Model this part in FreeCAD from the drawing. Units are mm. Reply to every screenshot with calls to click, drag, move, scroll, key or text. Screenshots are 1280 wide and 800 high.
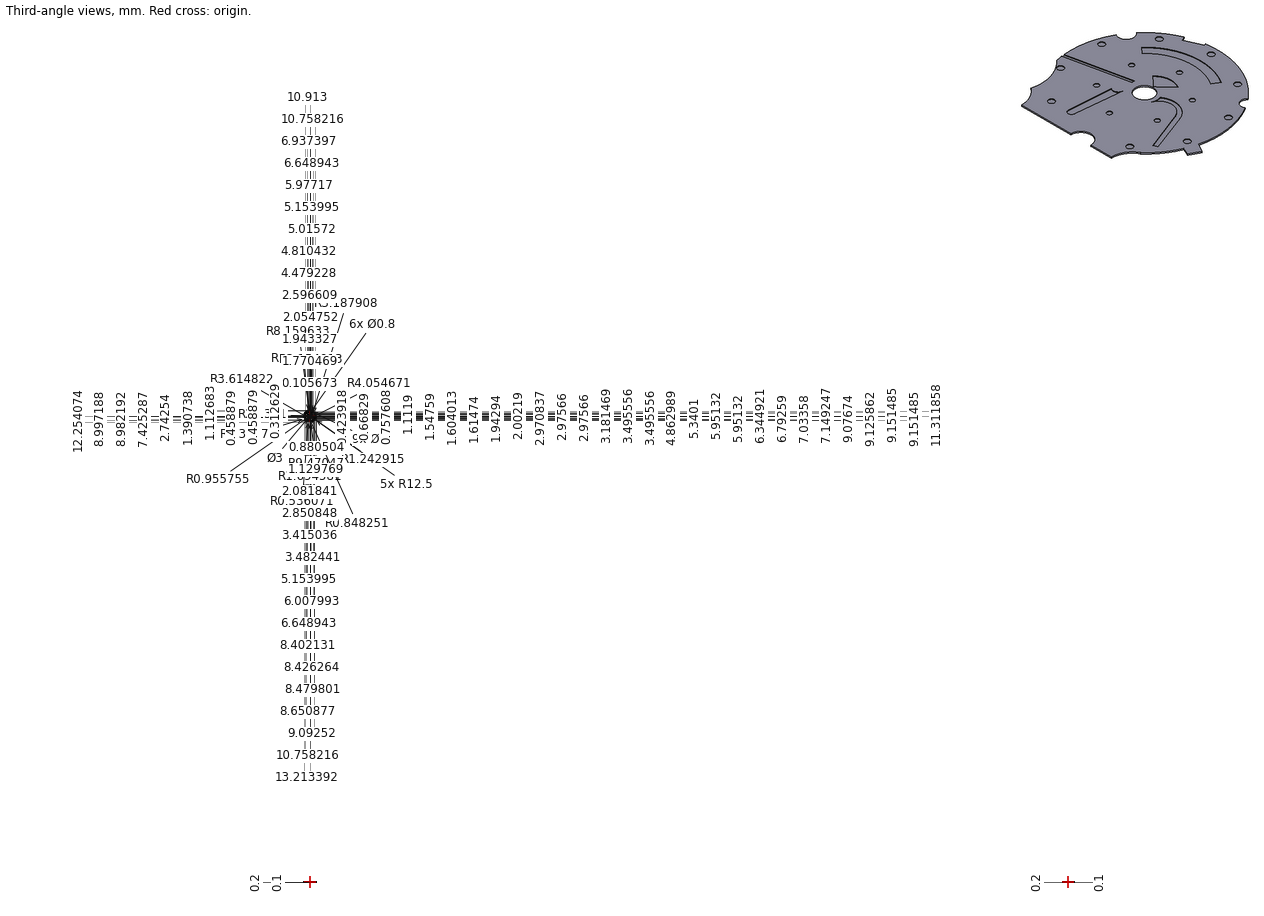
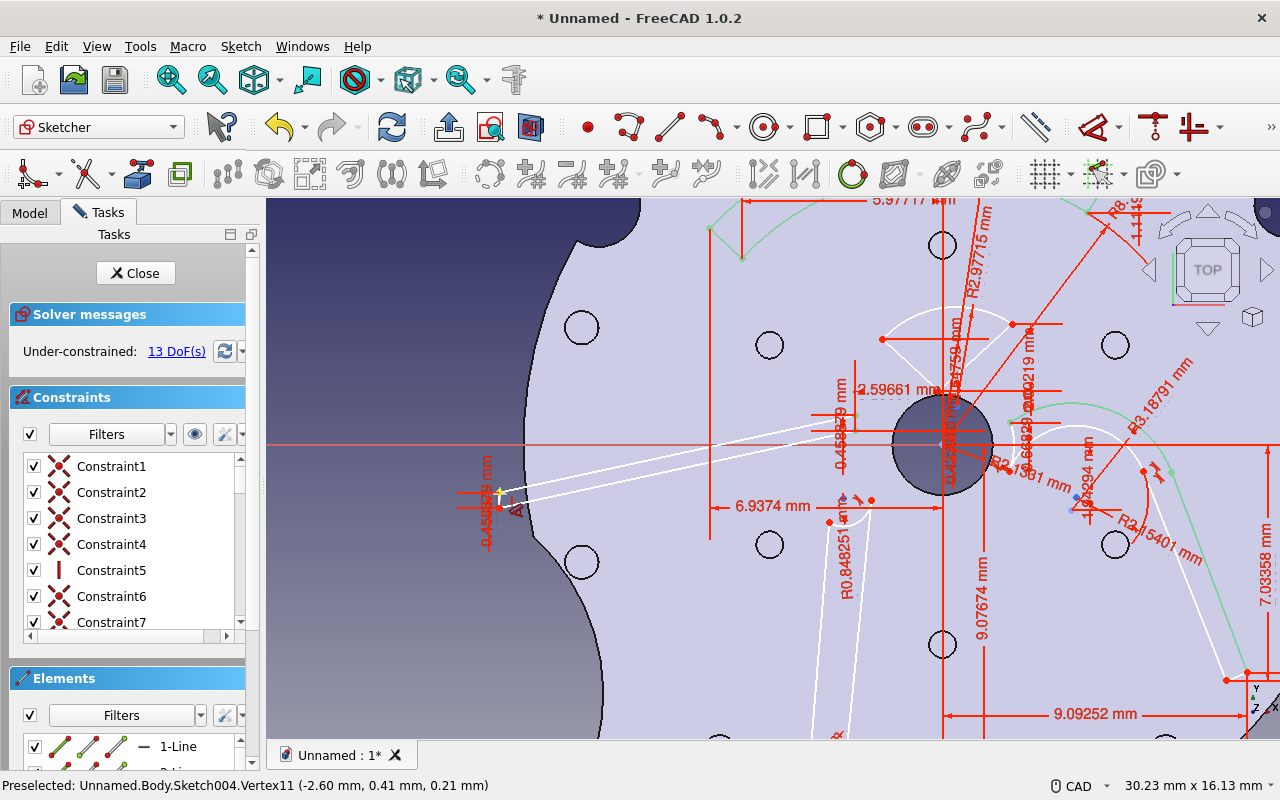
click(499, 493)
click(465, 469)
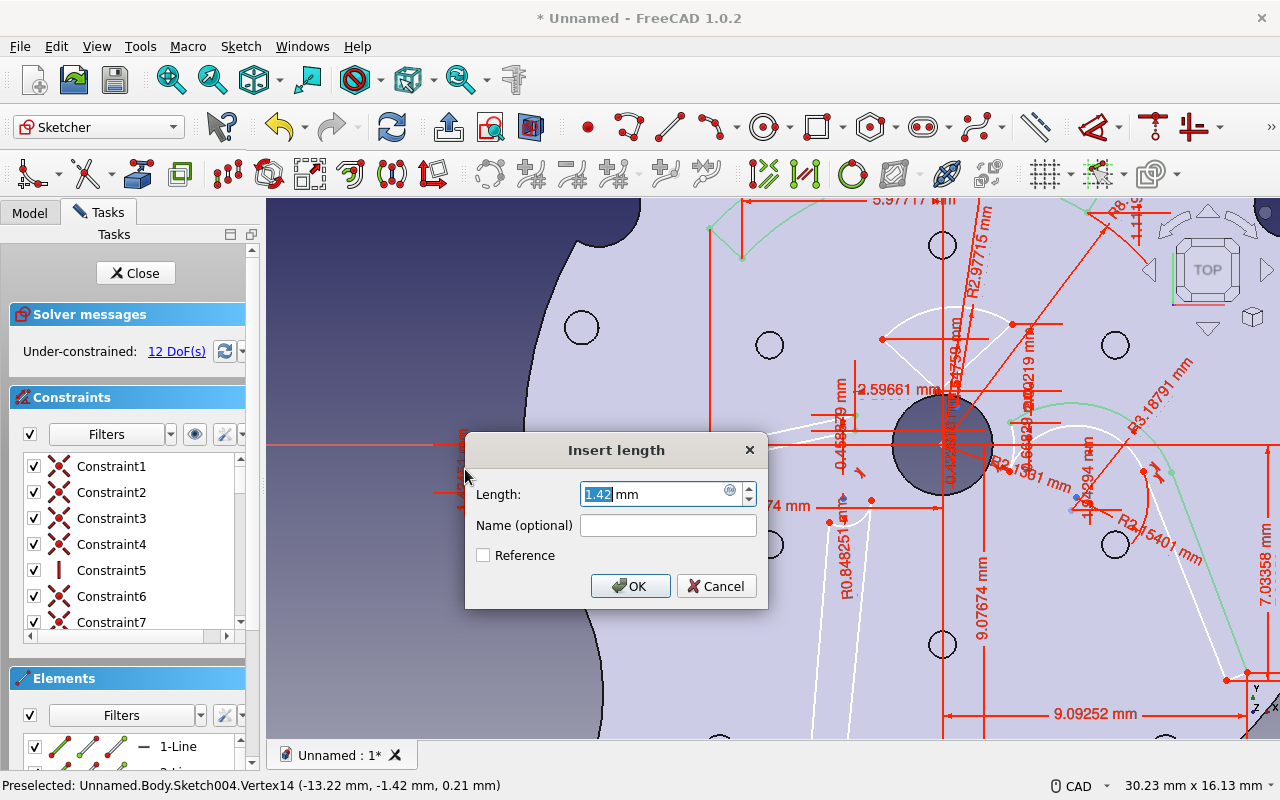
text(1.390738)
key(Return)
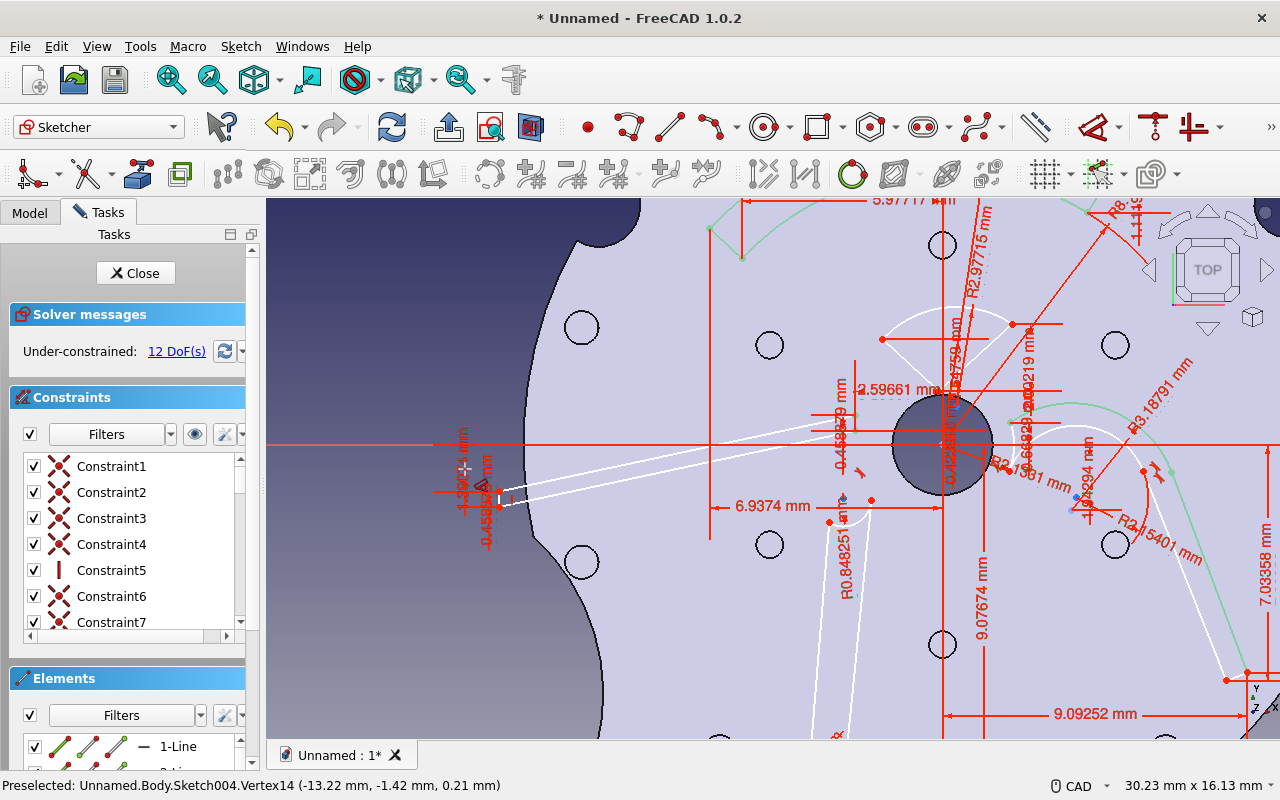
scroll(499, 493, down, 3)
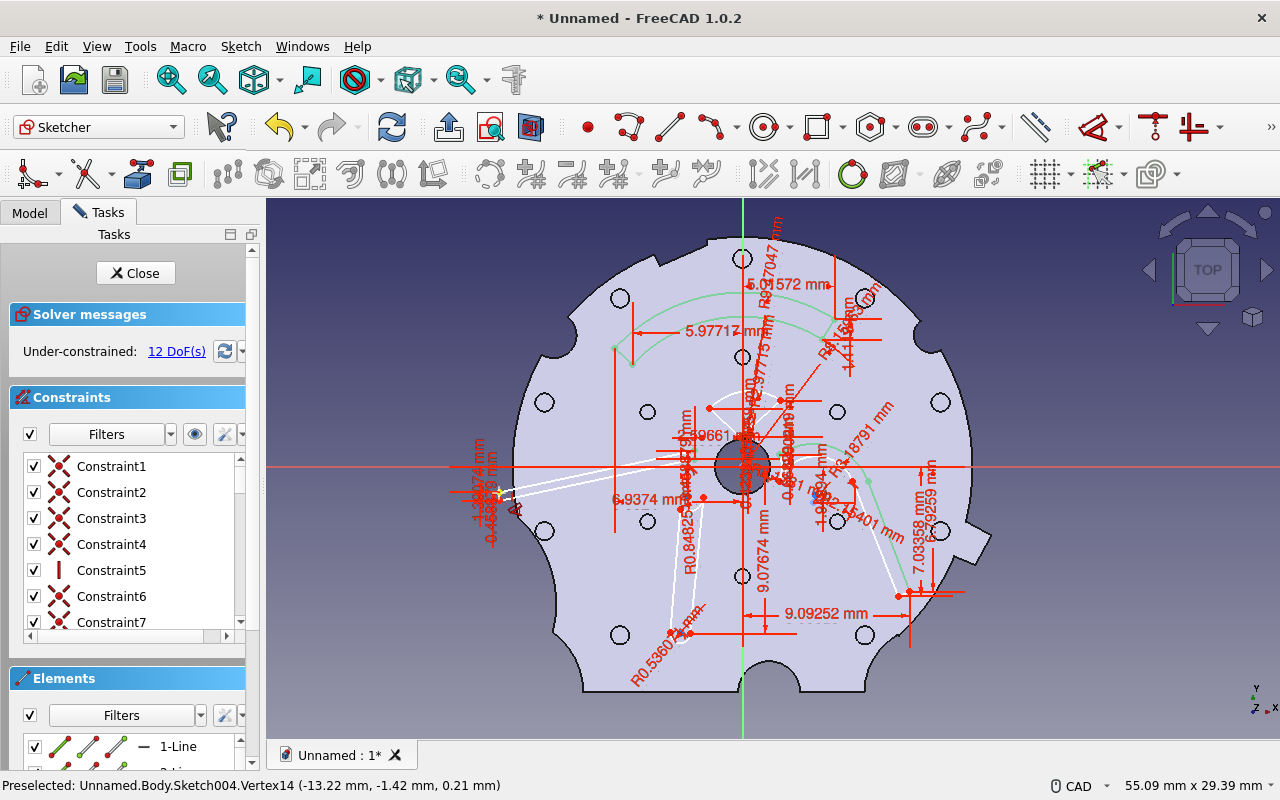
scroll(690, 634, up, 2)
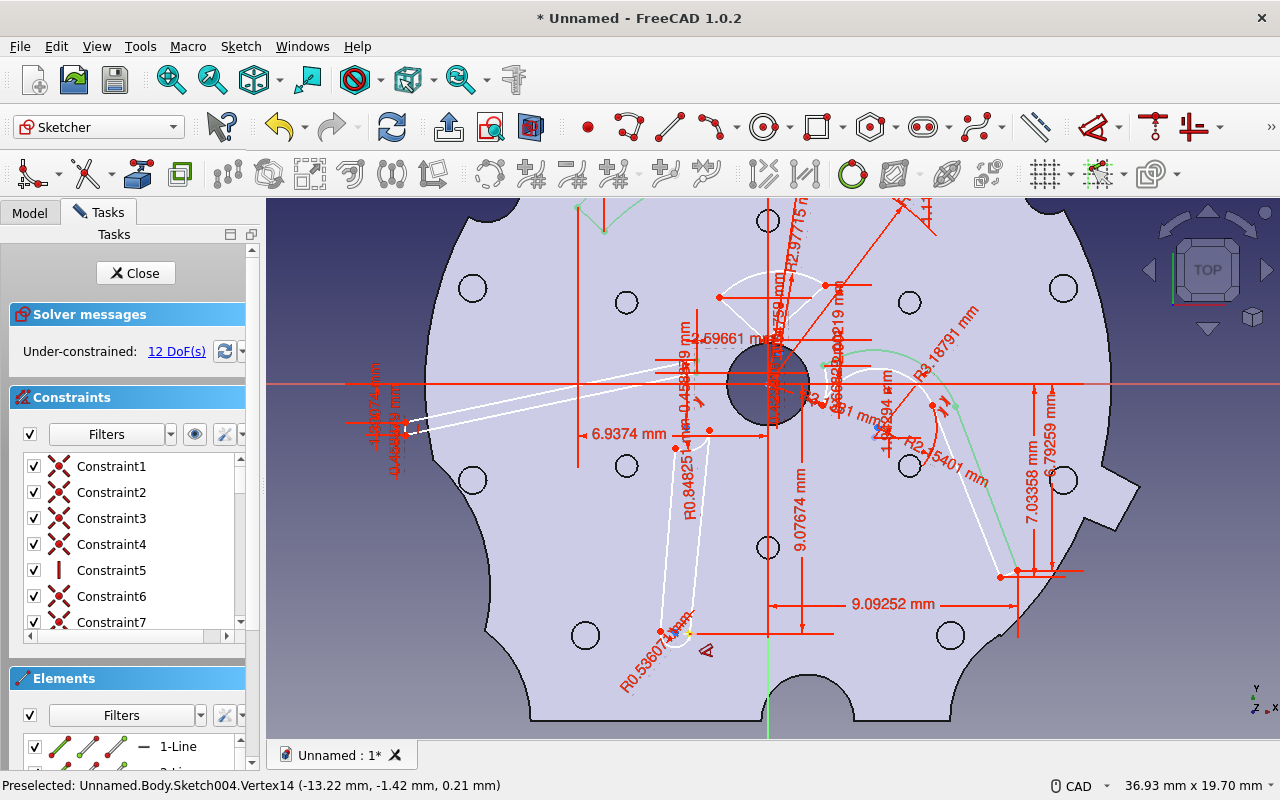
click(690, 634)
click(729, 668)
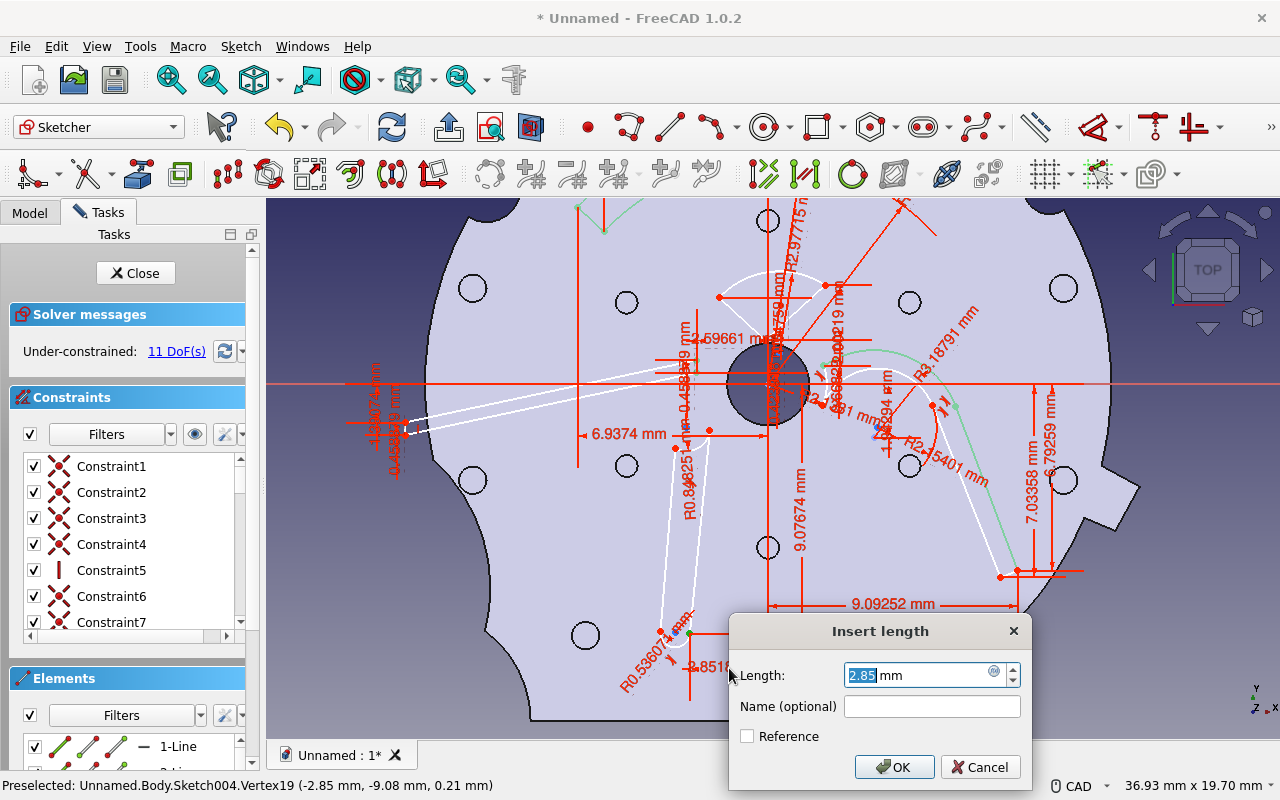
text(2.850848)
key(Return)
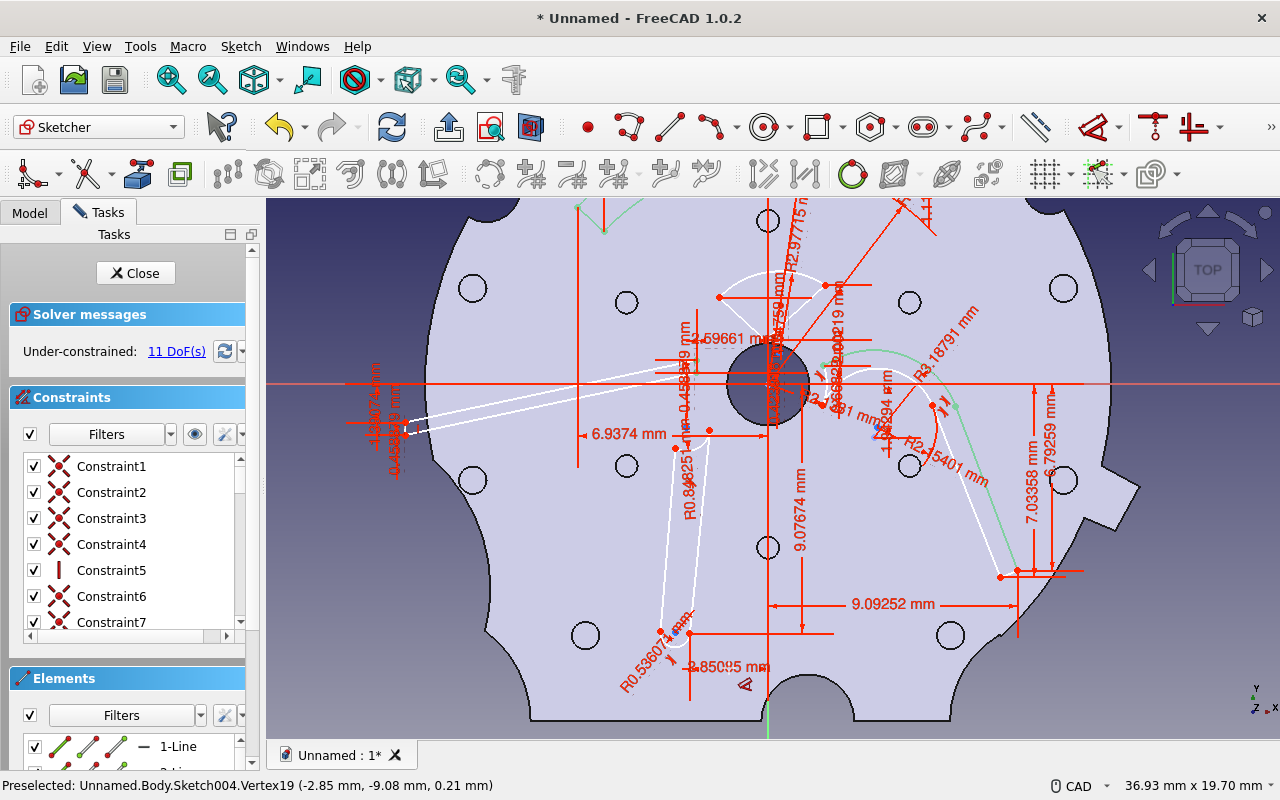
click(710, 430)
click(726, 512)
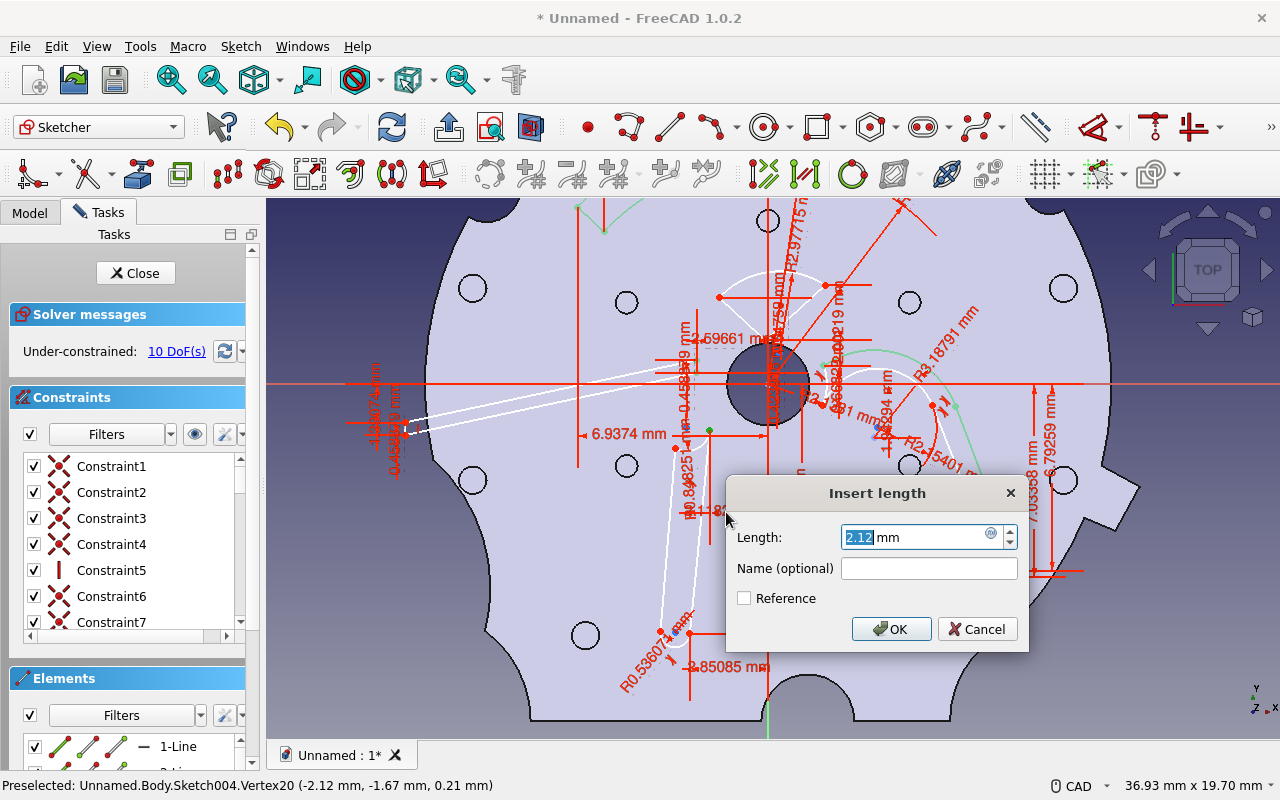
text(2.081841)
key(Return)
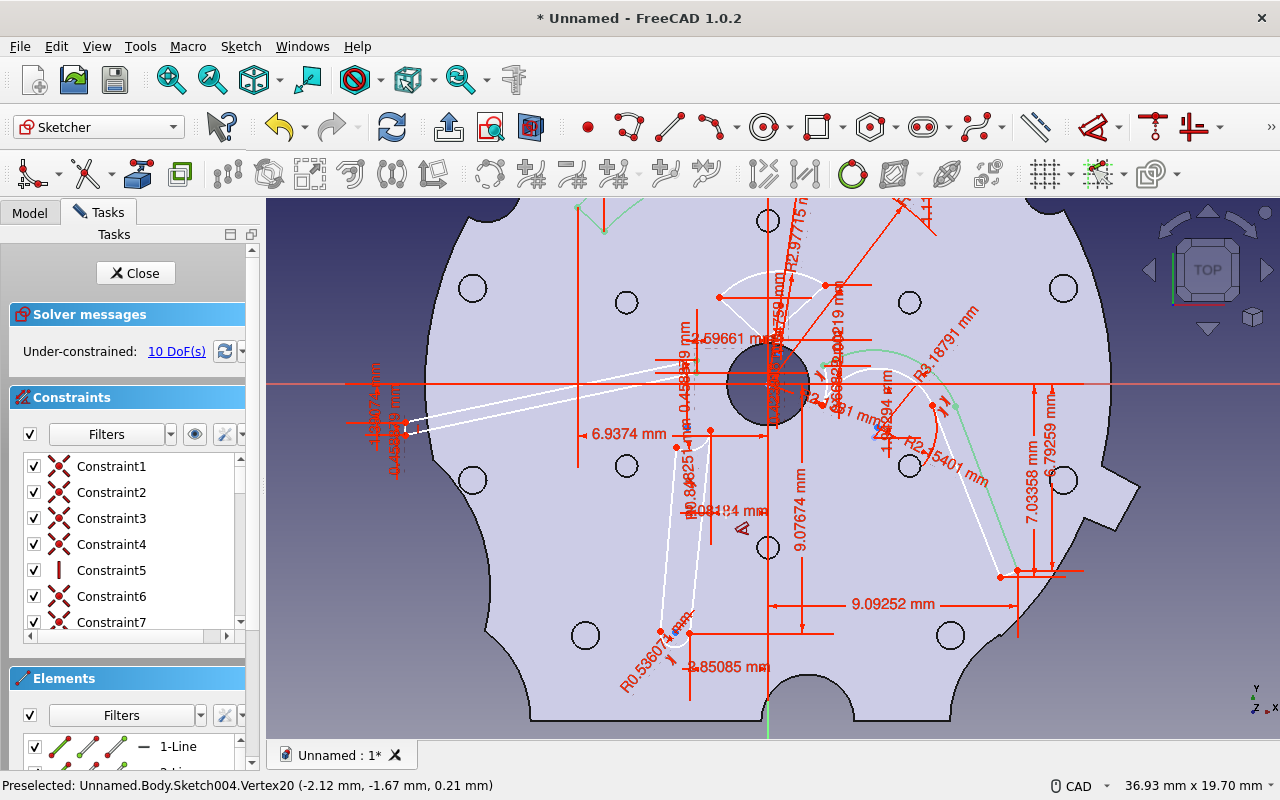
click(711, 430)
click(677, 407)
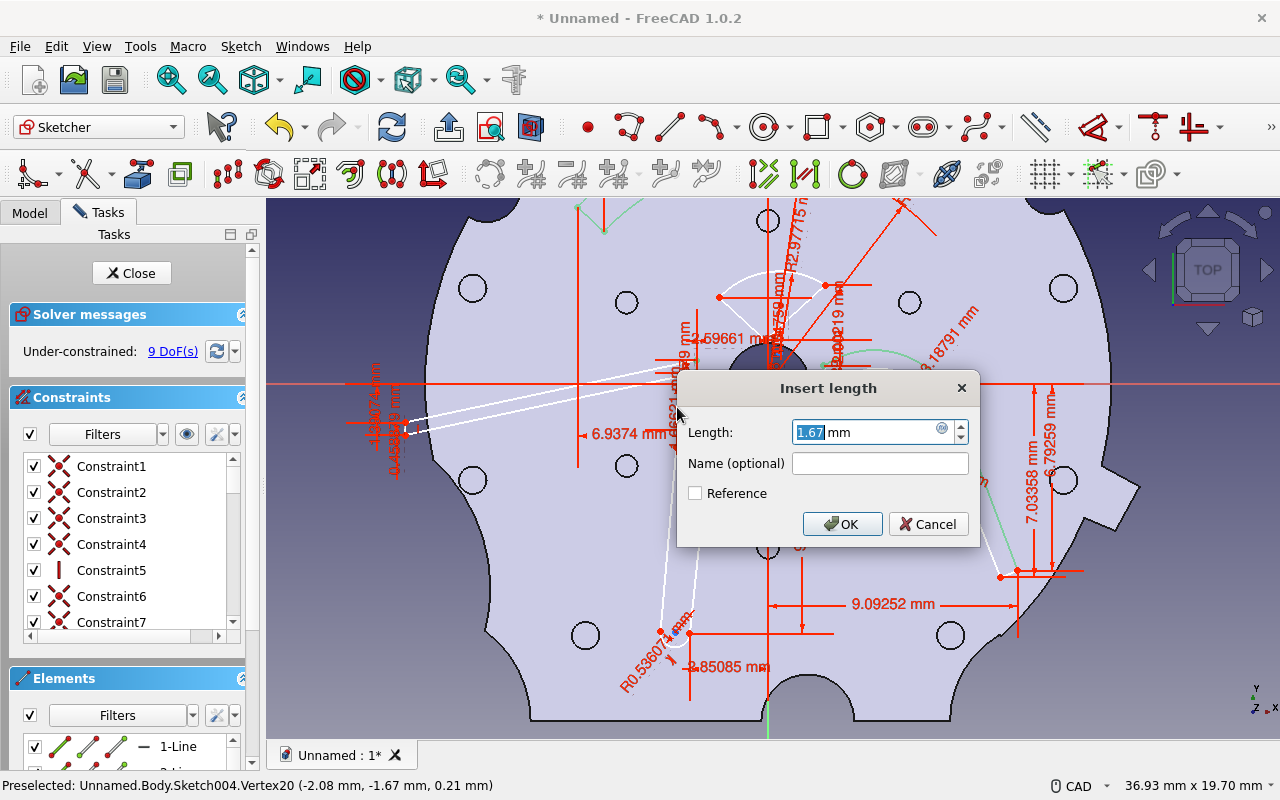
text(1.604013)
key(Return)